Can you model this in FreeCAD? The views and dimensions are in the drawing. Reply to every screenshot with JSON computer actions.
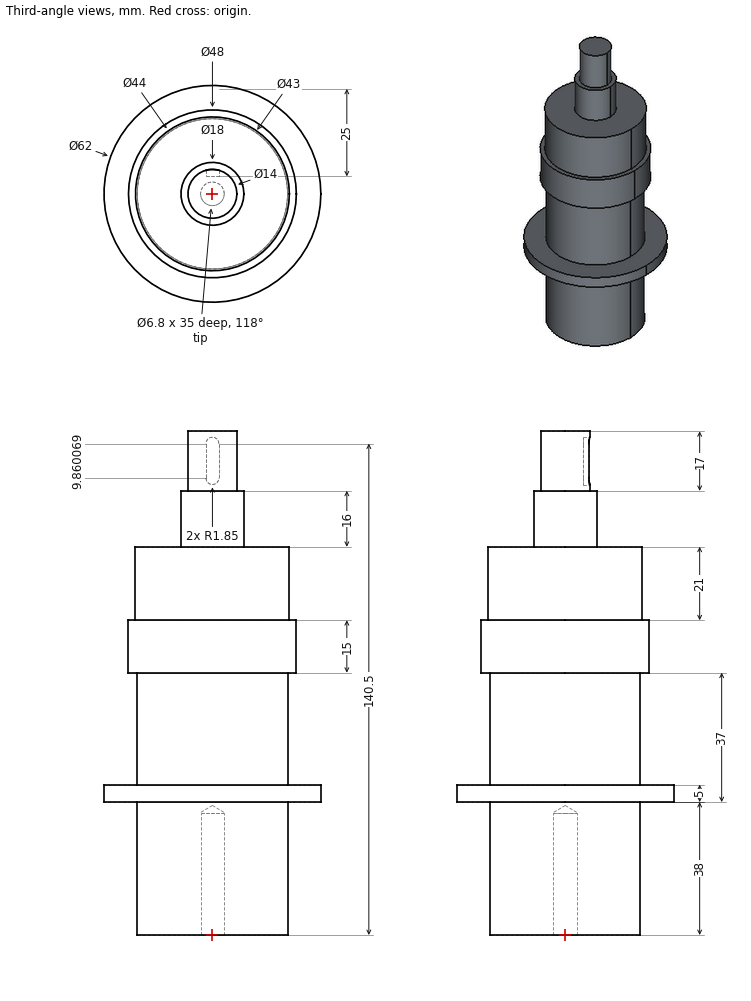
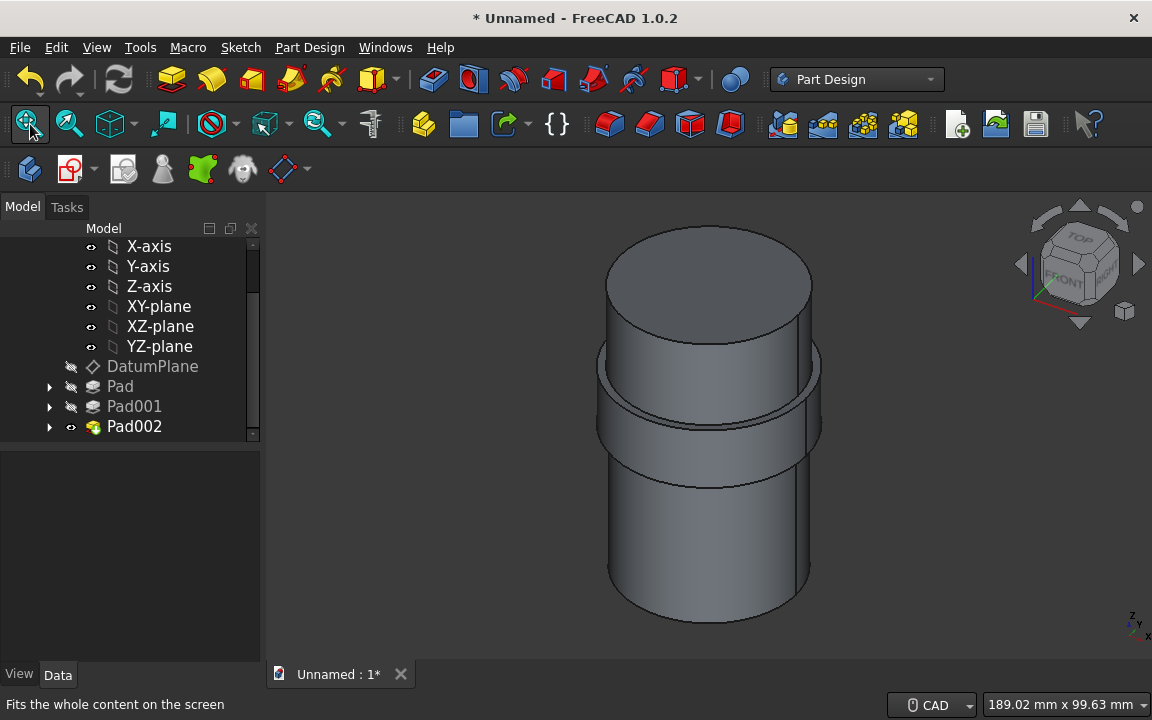
{"action": "left_click", "coordinate": [709, 284]}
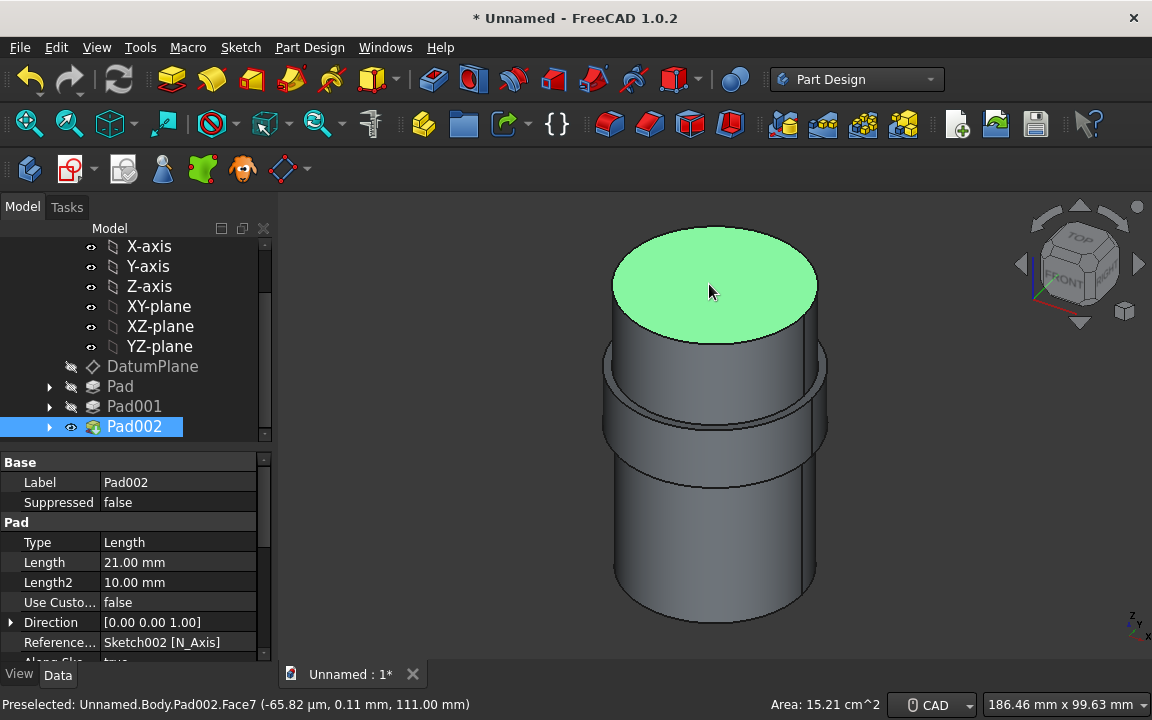
{"action": "left_click", "coordinate": [70, 170]}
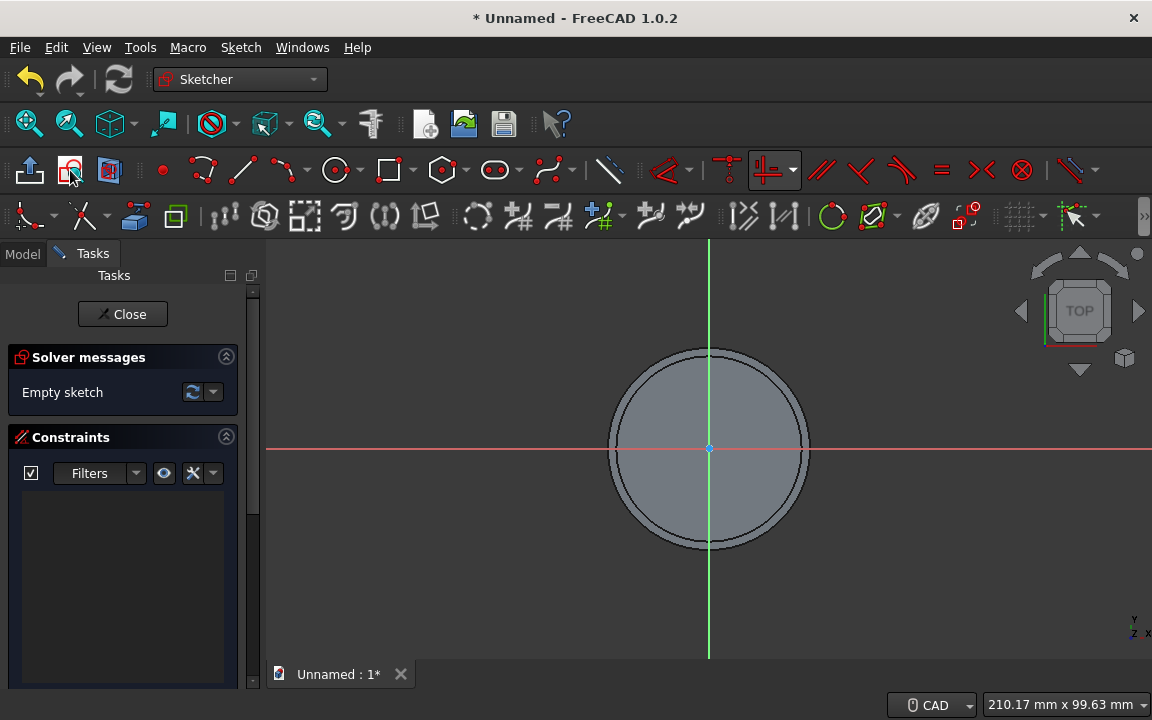
{"action": "scroll", "coordinate": [739, 449], "scroll_direction": "up", "scroll_amount": 6}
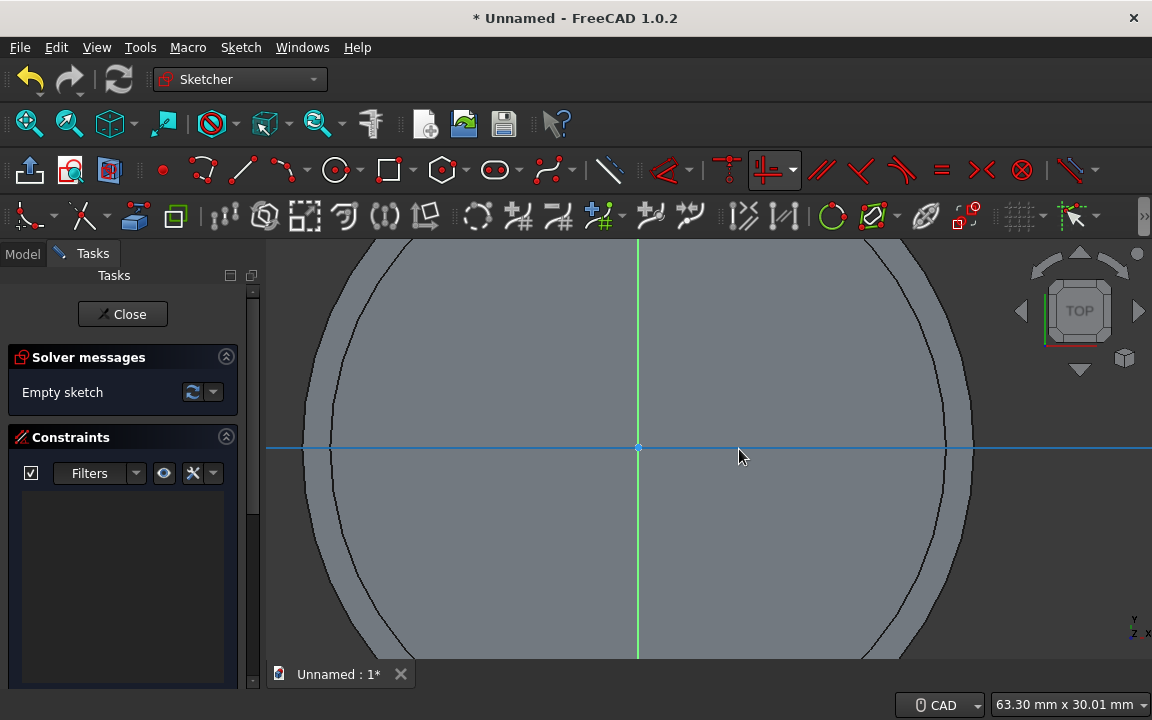
{"action": "left_click", "coordinate": [336, 170]}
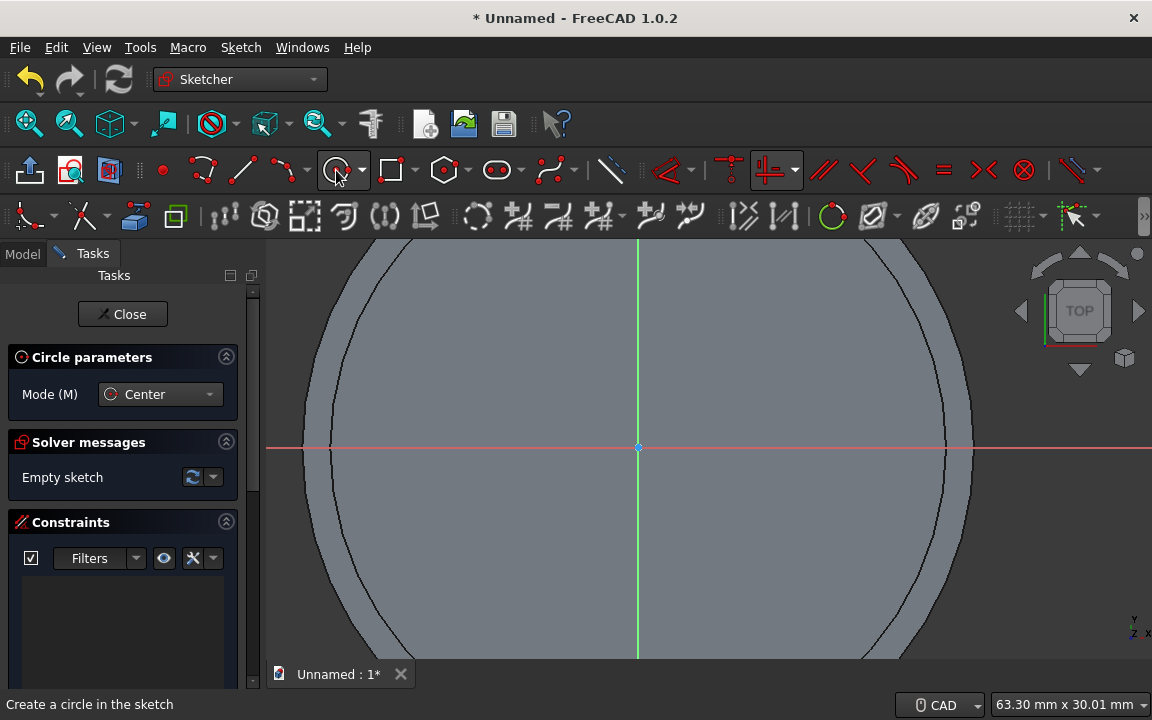
{"action": "left_click", "coordinate": [638, 448]}
{"action": "left_click", "coordinate": [727, 359]}
{"action": "key", "text": "Escape"}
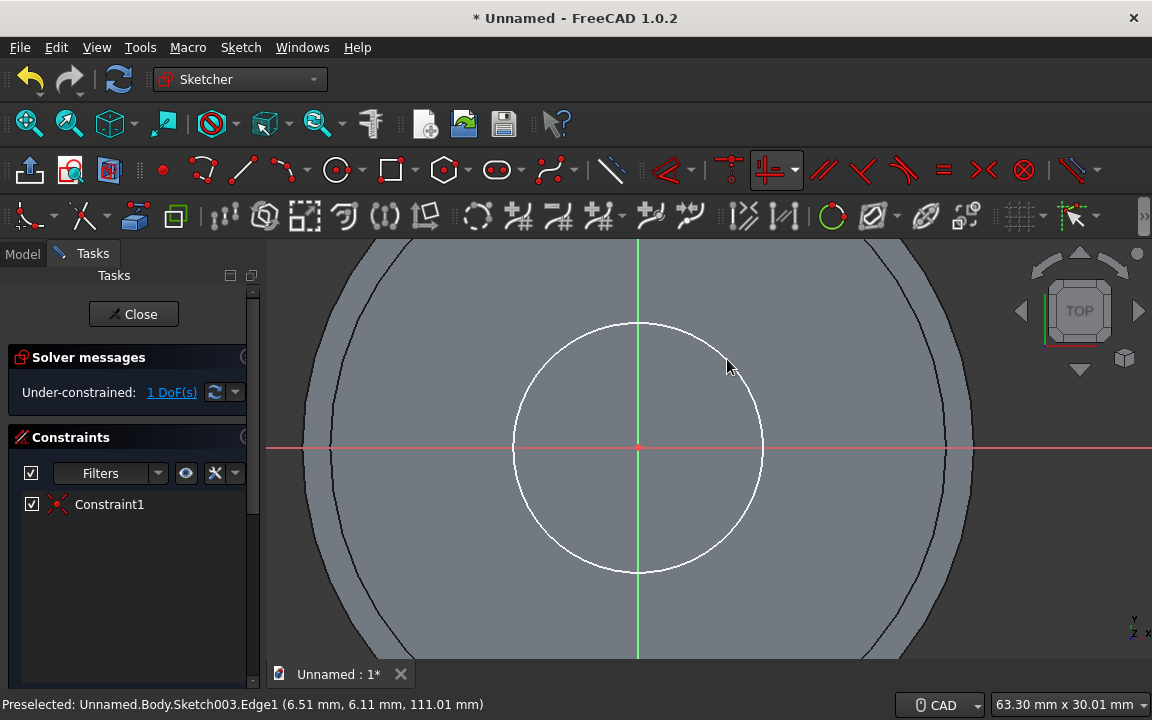
{"action": "key", "text": "d"}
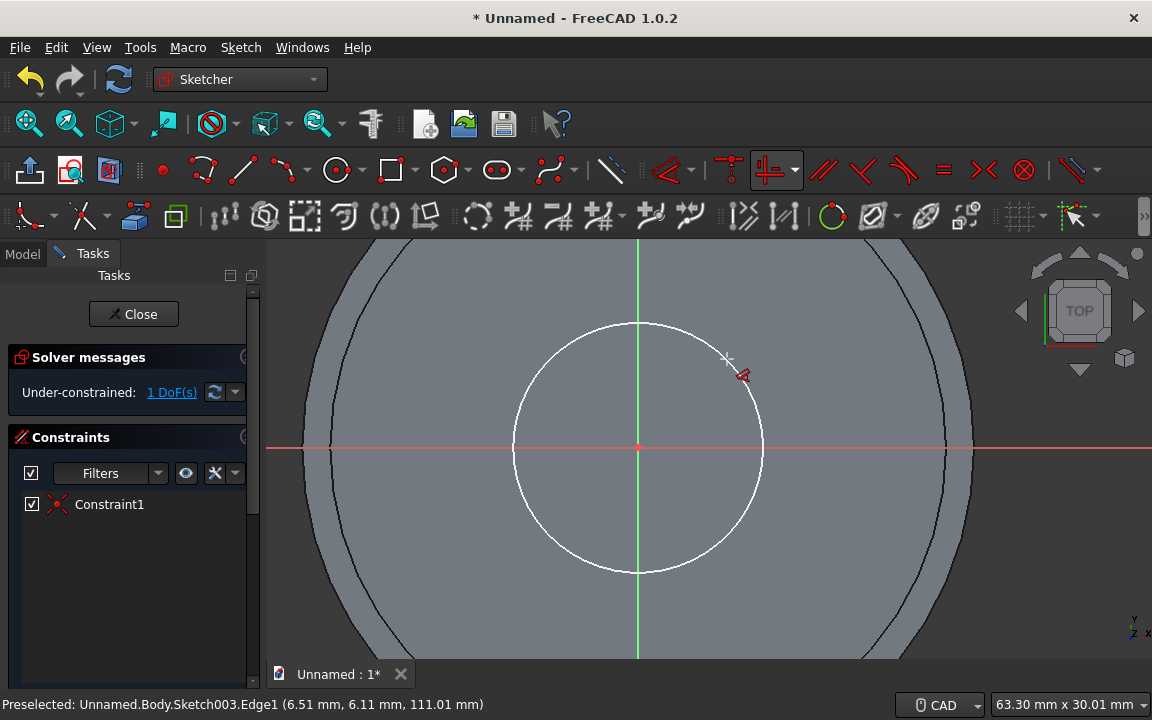
{"action": "left_click", "coordinate": [726, 359]}
{"action": "left_click", "coordinate": [748, 336]}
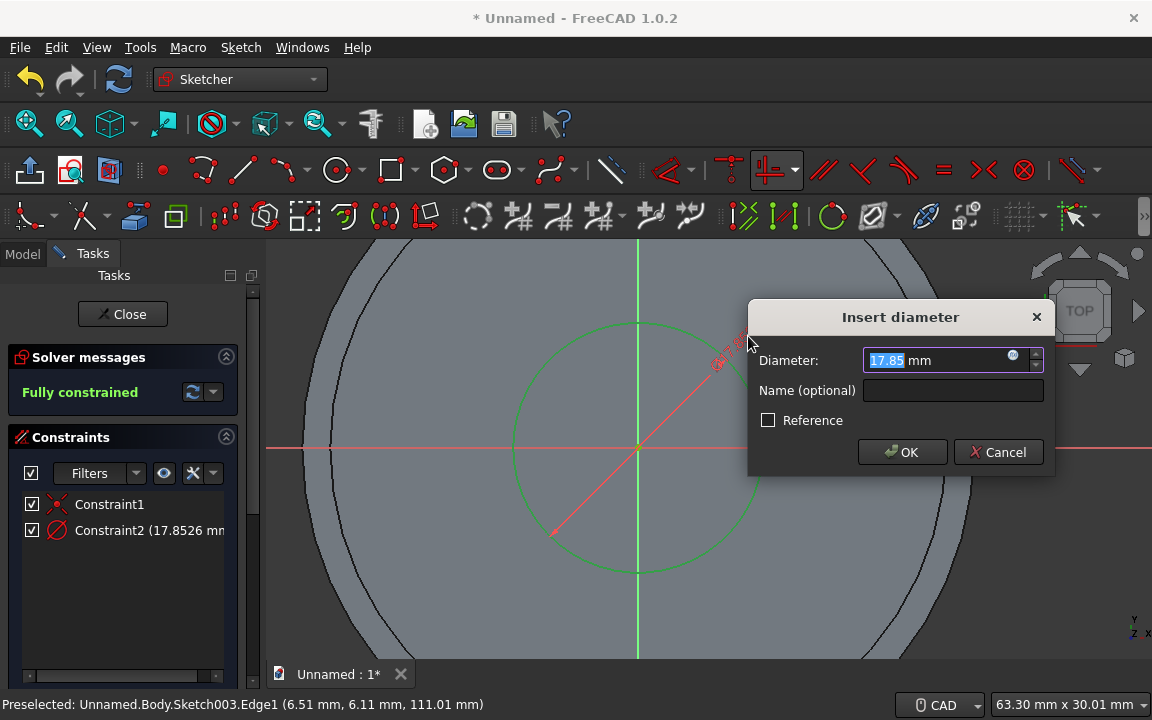
{"action": "type", "text": "18"}
{"action": "key", "text": "Return"}
{"action": "key", "text": "Escape"}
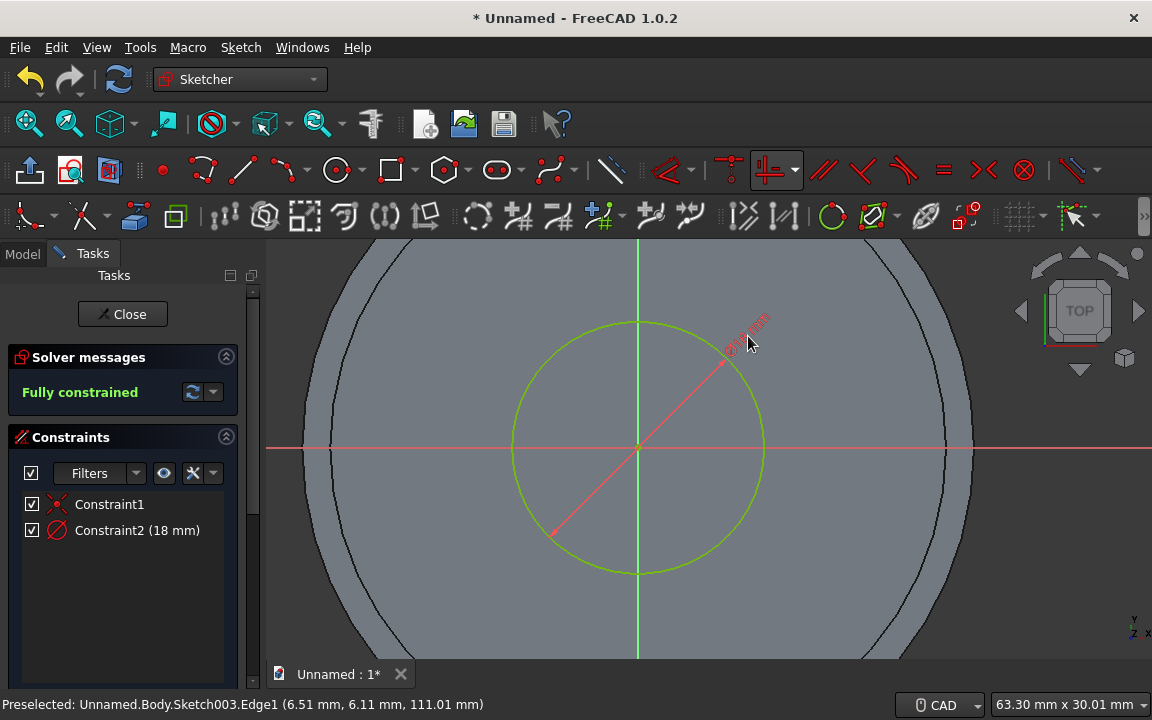
{"action": "left_click", "coordinate": [123, 314]}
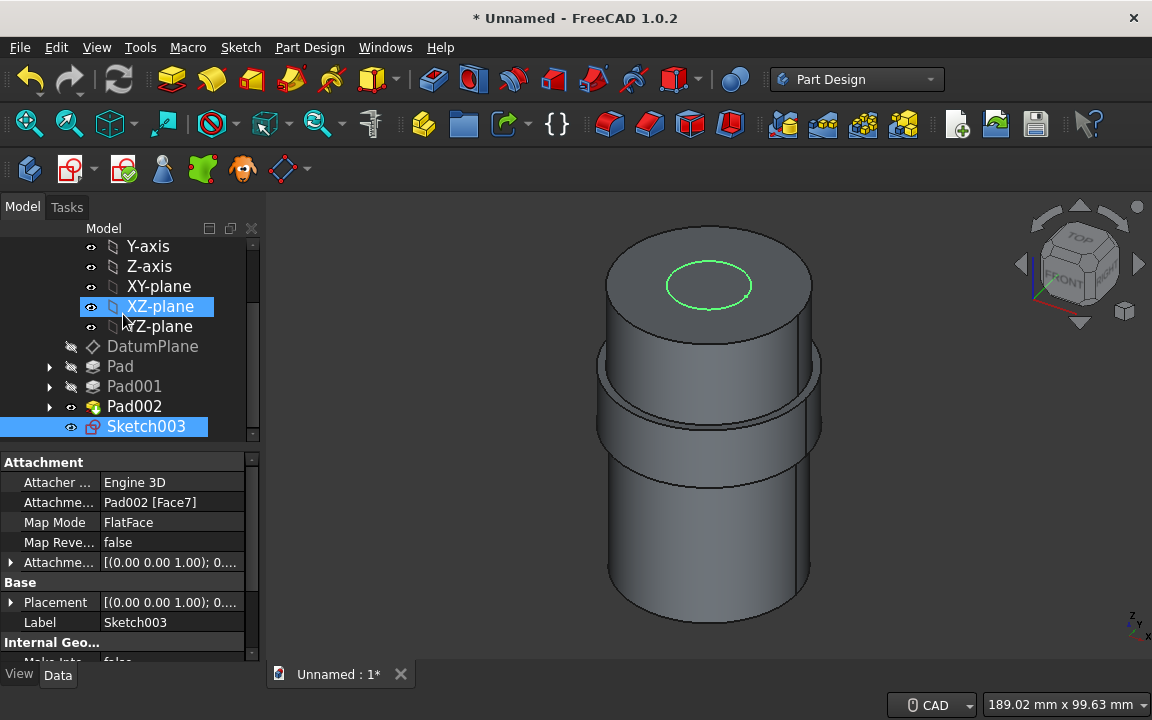
{"action": "left_click", "coordinate": [172, 80]}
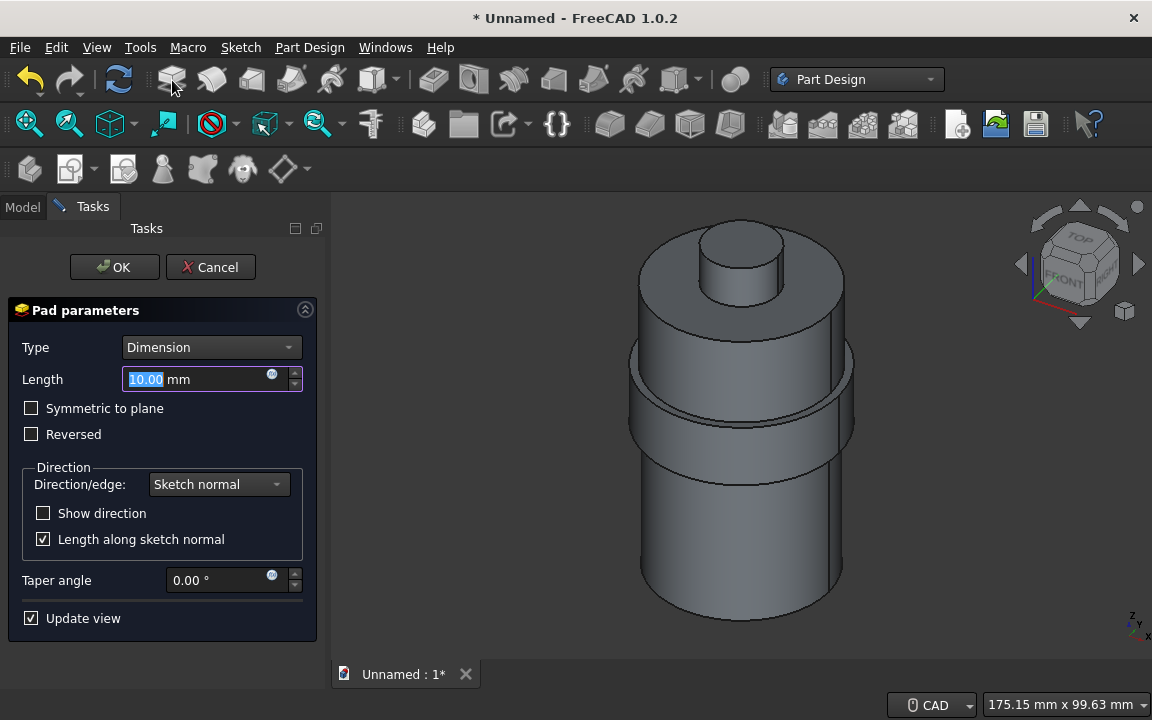
{"action": "type", "text": "16"}
{"action": "key", "text": "Tab"}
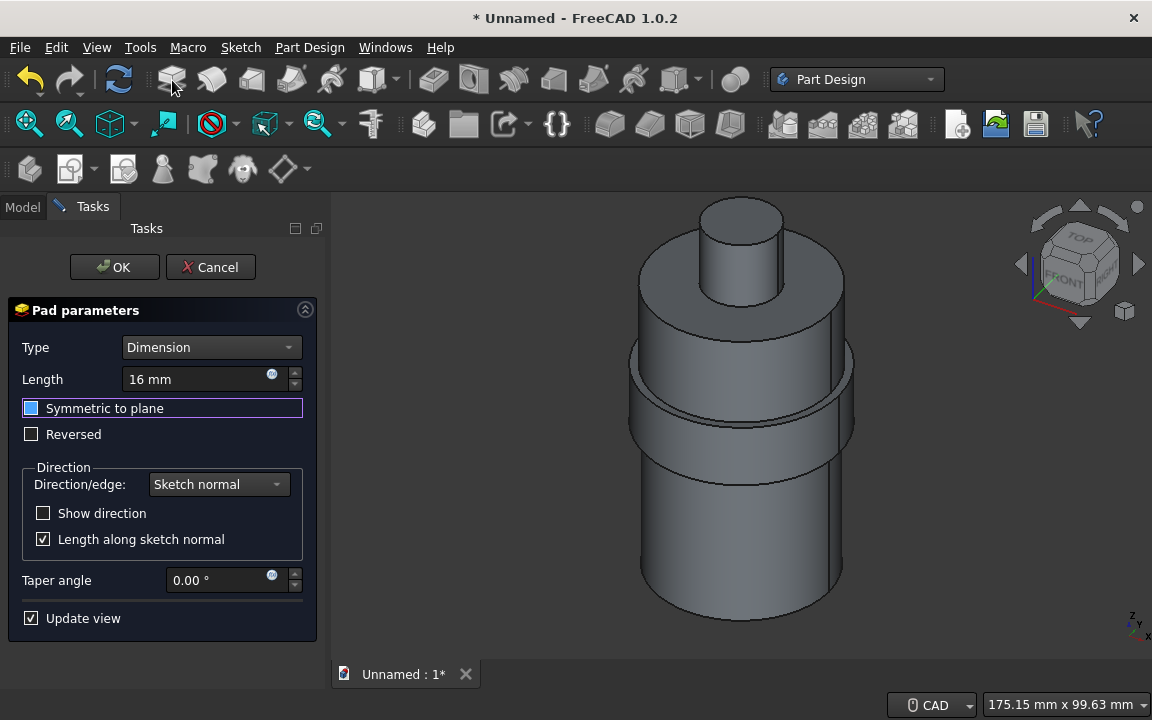
{"action": "left_click", "coordinate": [115, 267]}